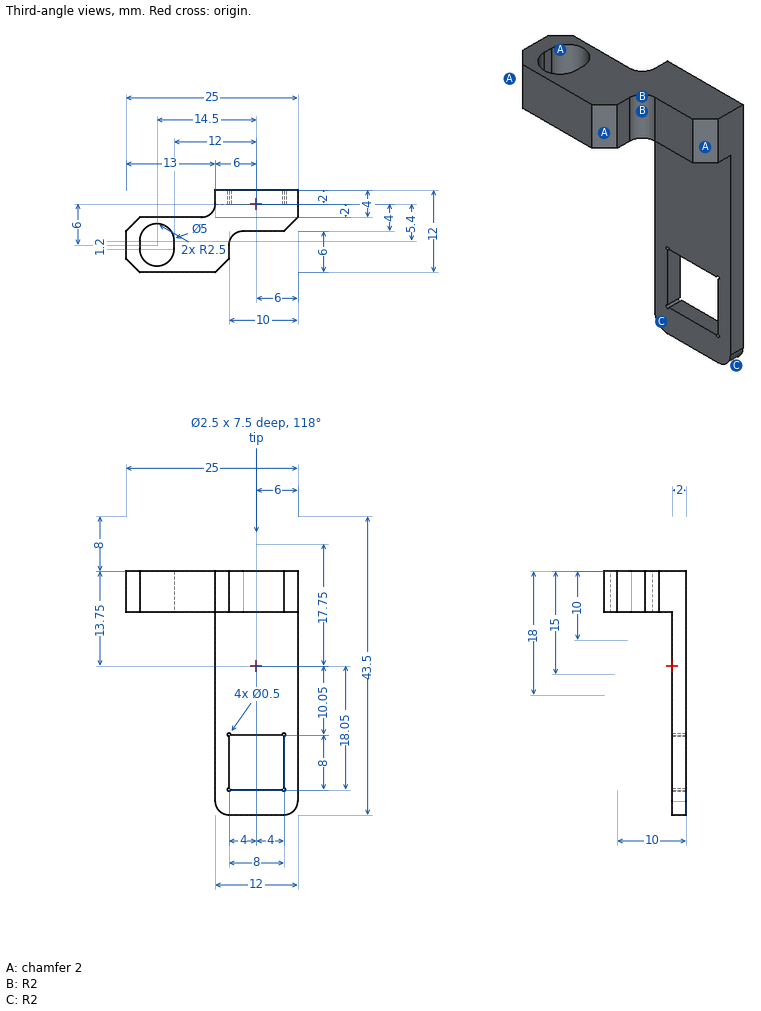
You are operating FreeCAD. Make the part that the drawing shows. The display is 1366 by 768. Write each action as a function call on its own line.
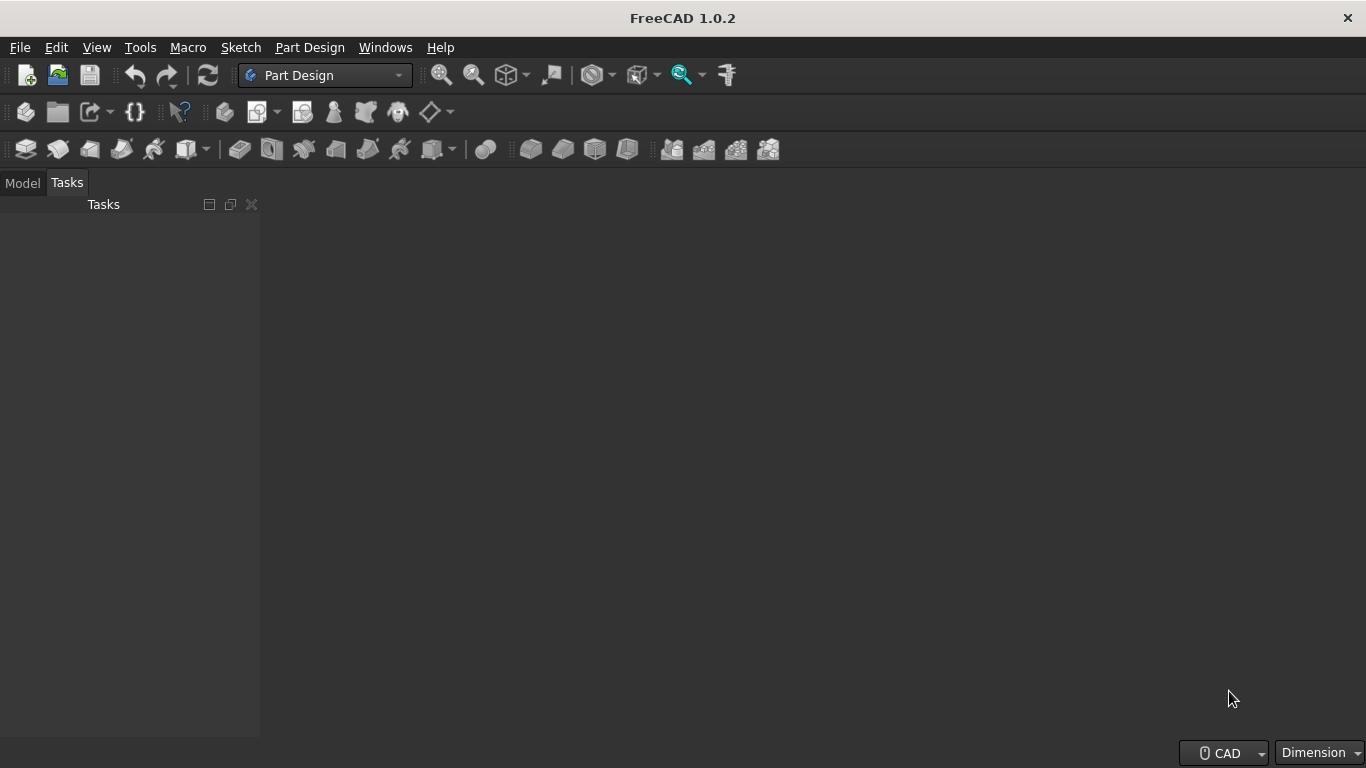
click(26, 76)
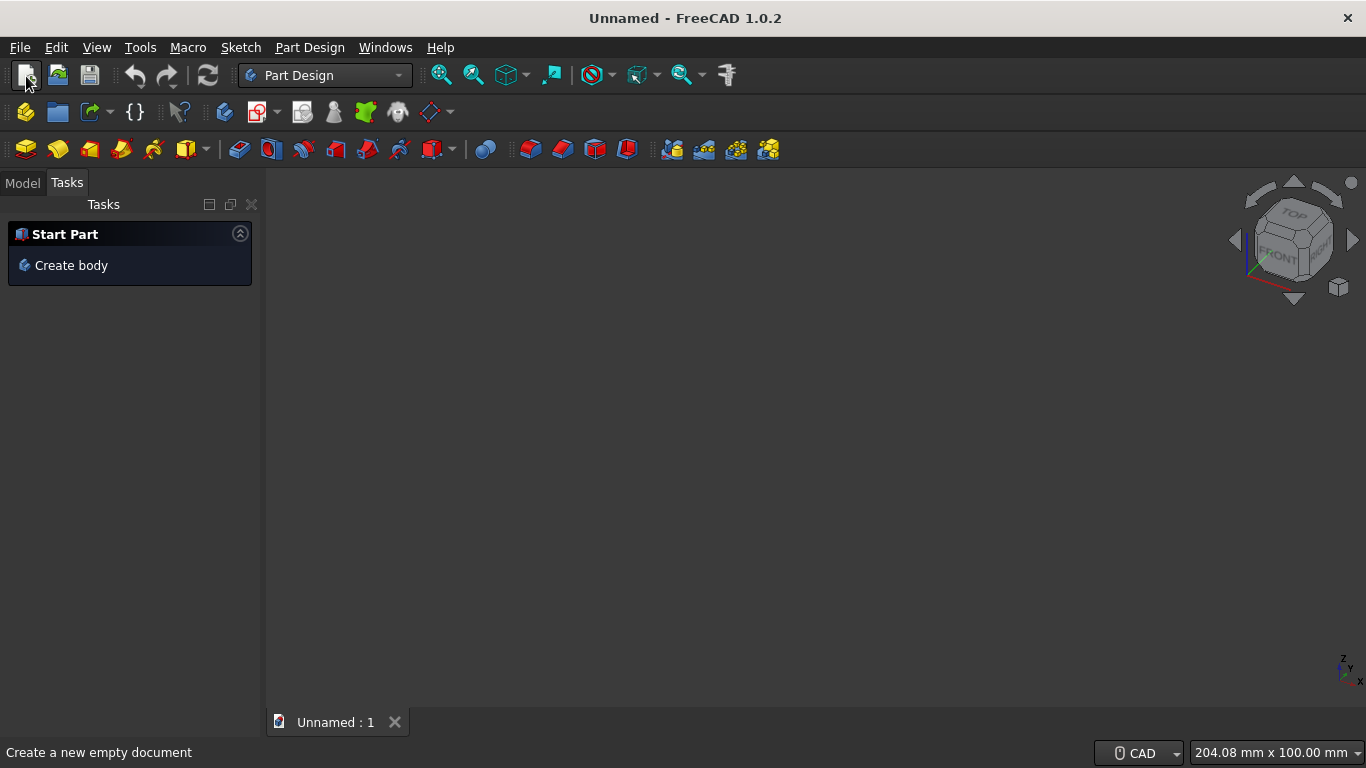
click(258, 112)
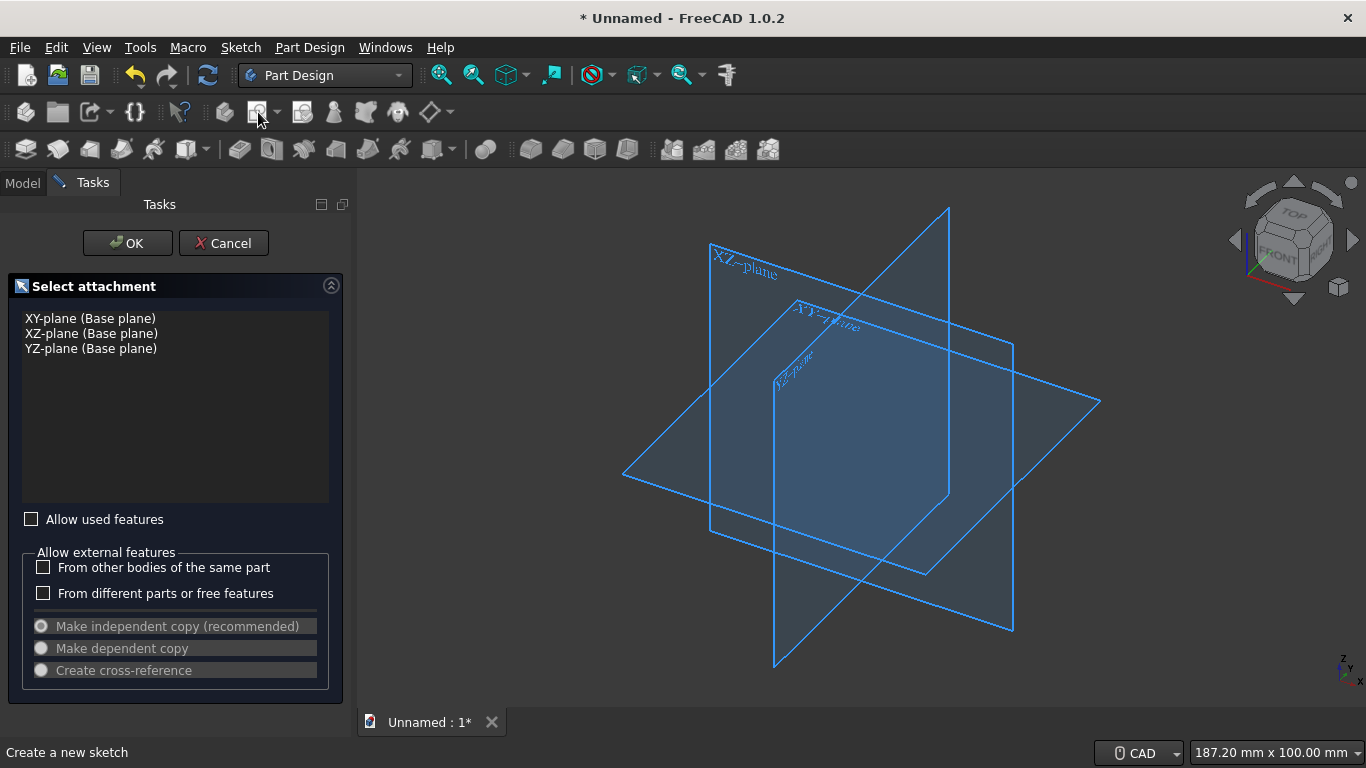
click(82, 334)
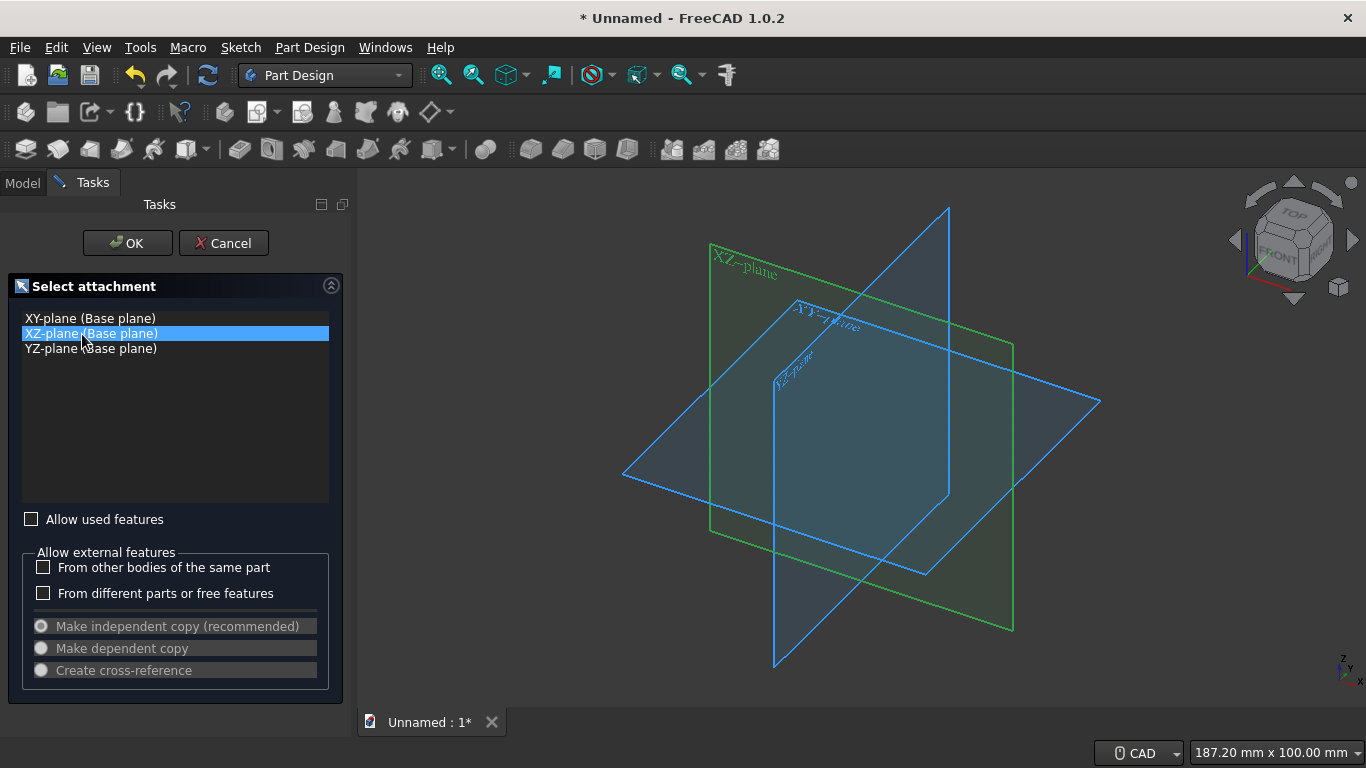
click(128, 243)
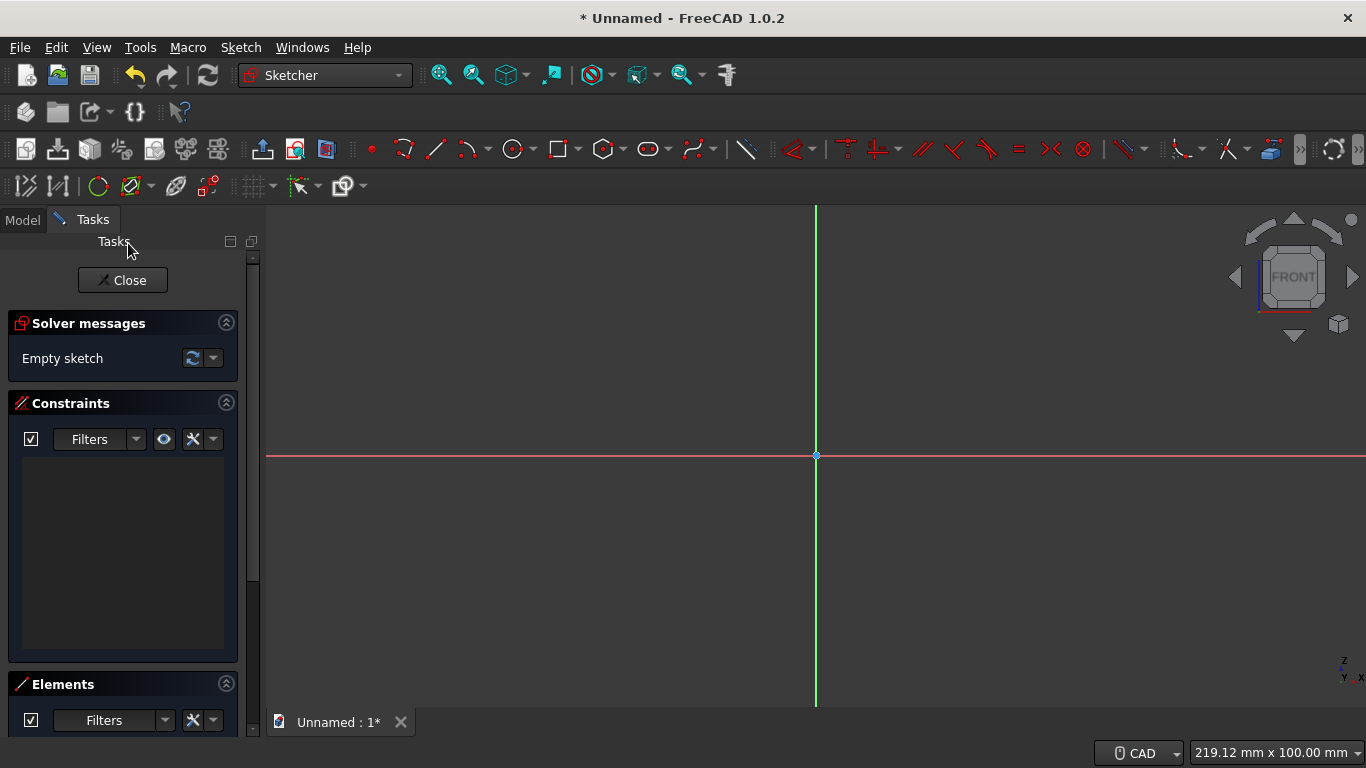
scroll(955, 456, up, 2)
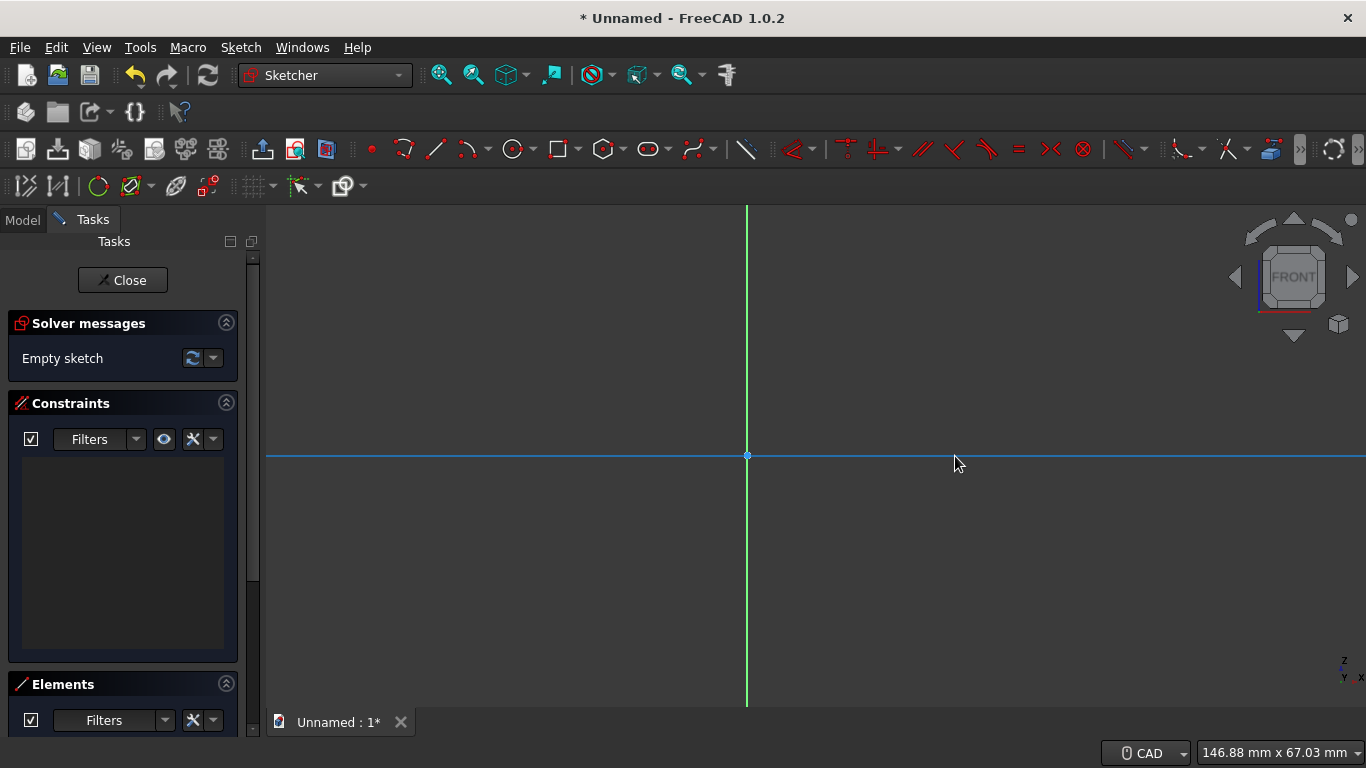
click(580, 150)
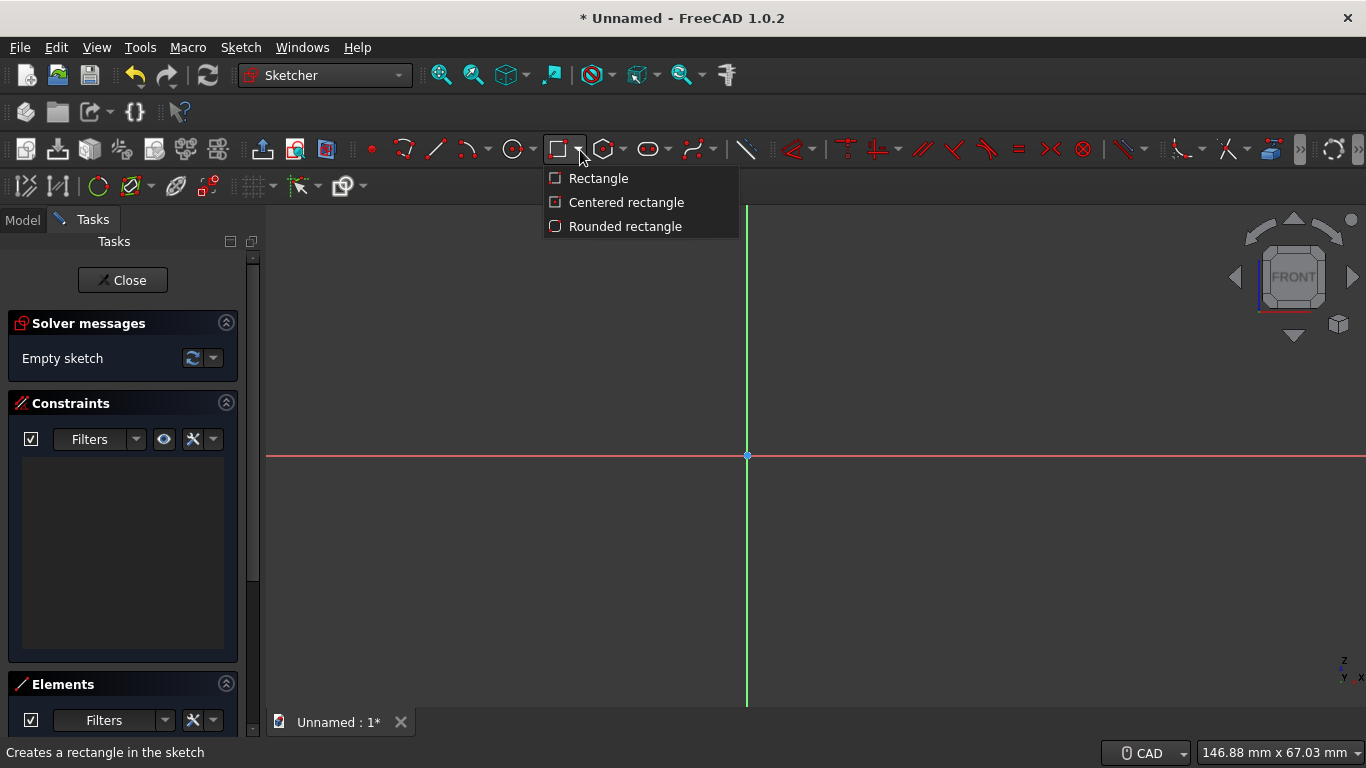
click(642, 202)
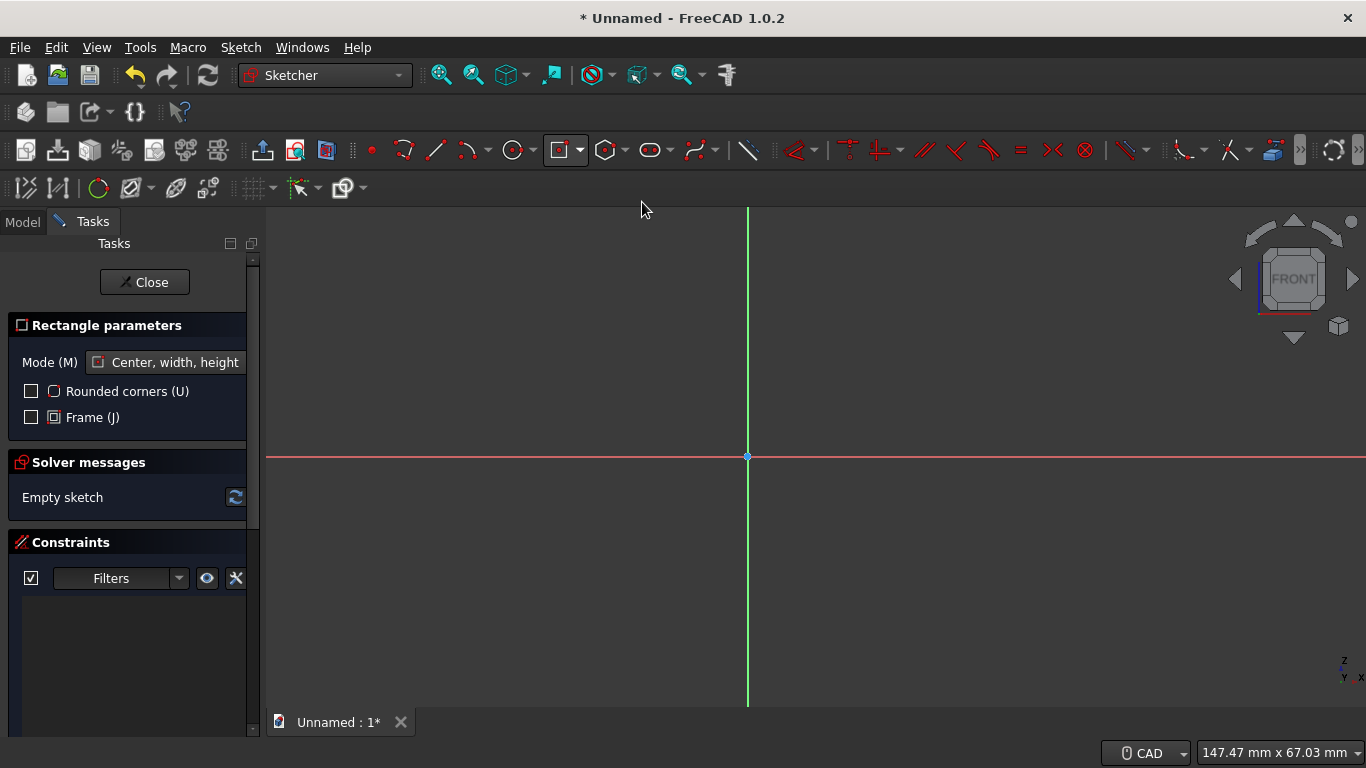
click(748, 457)
click(792, 295)
key(Escape)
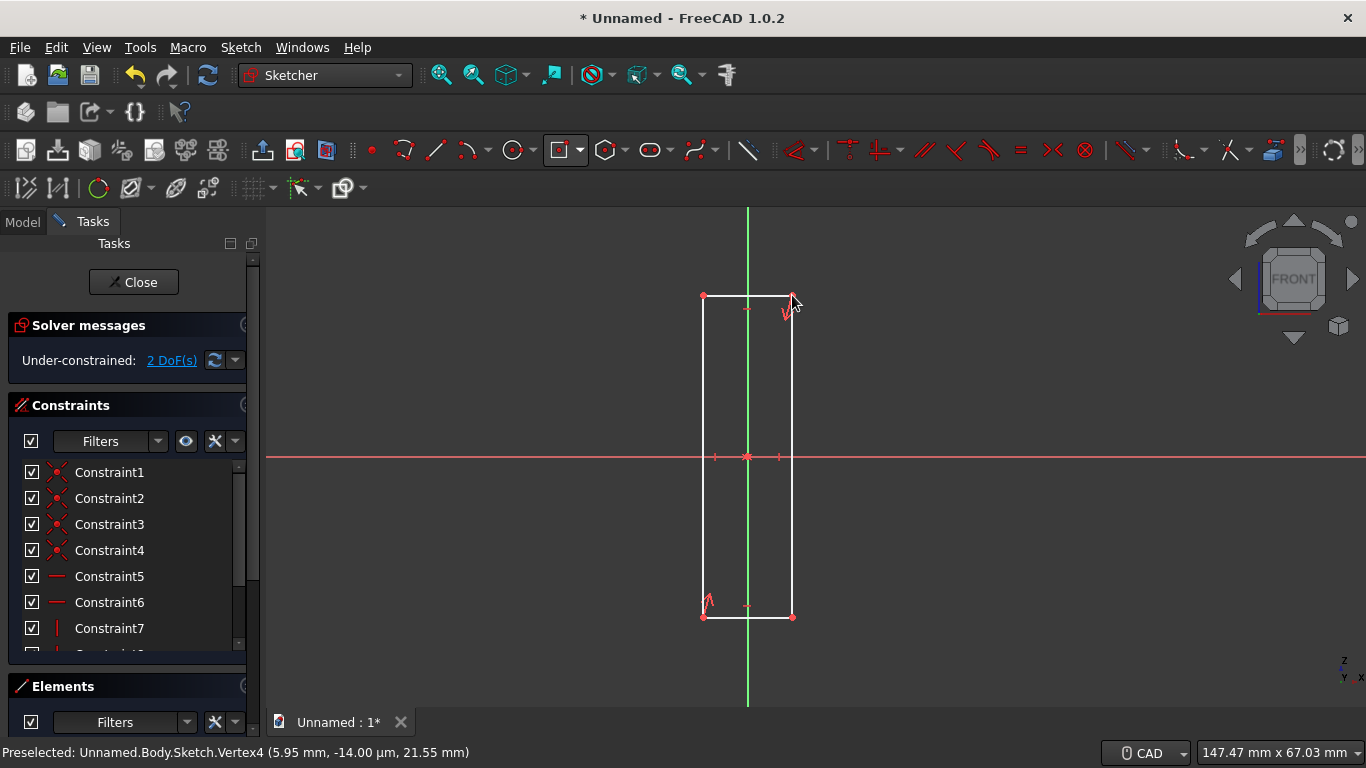
click(794, 150)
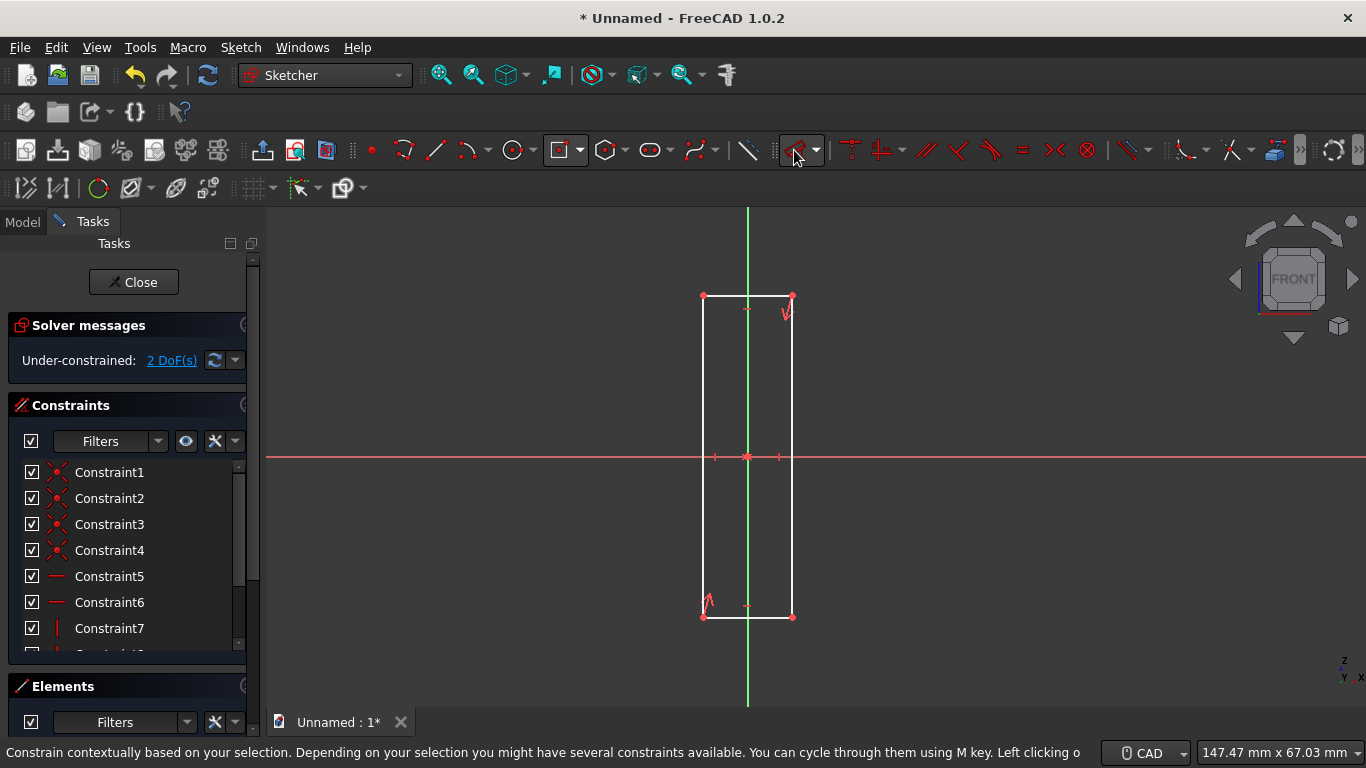
click(730, 618)
click(727, 652)